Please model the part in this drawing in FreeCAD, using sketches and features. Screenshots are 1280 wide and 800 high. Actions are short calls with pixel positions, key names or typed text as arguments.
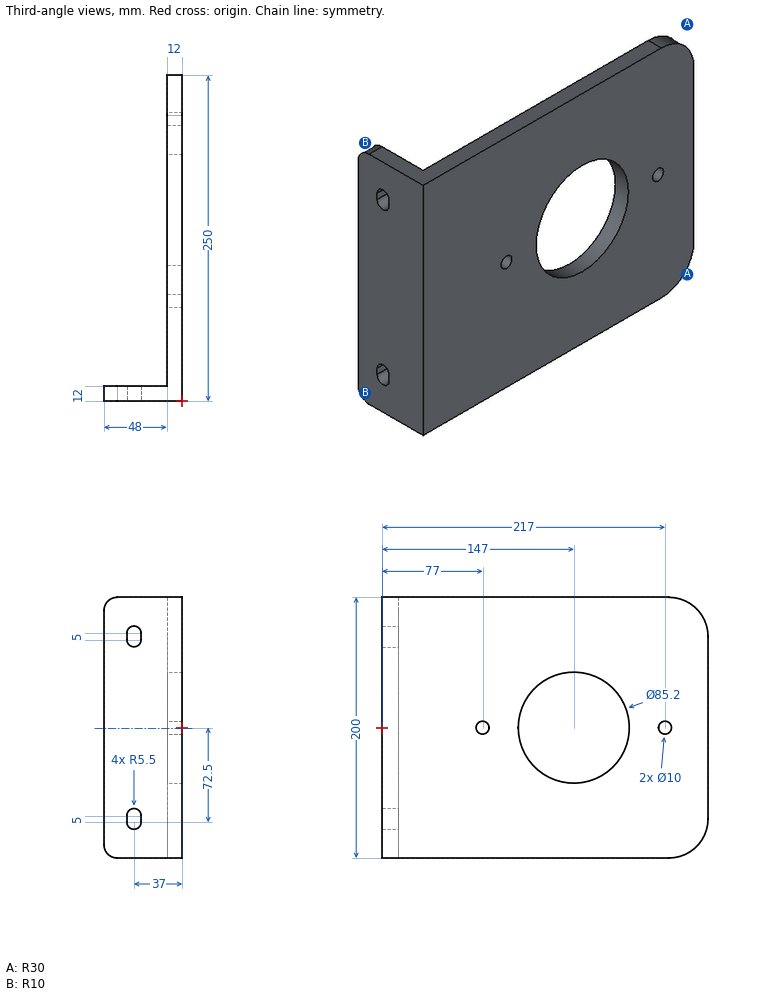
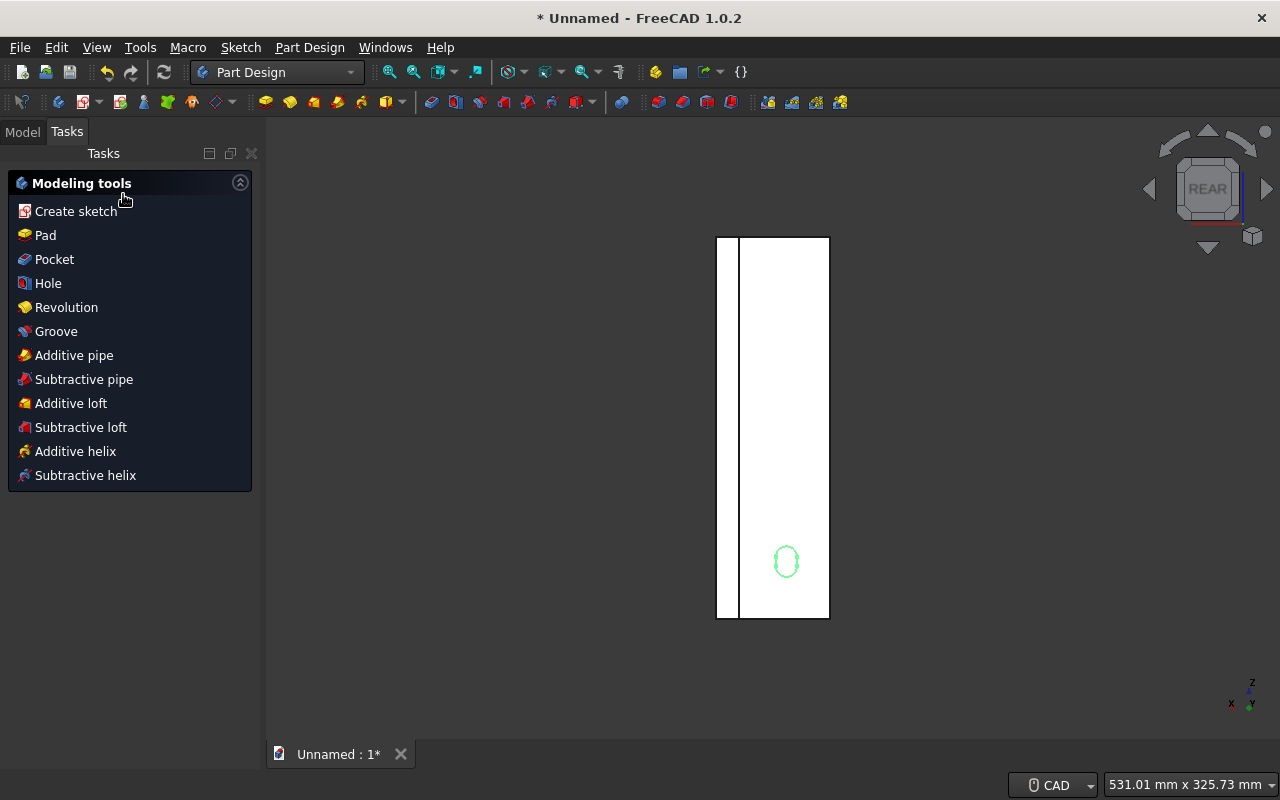
click(432, 102)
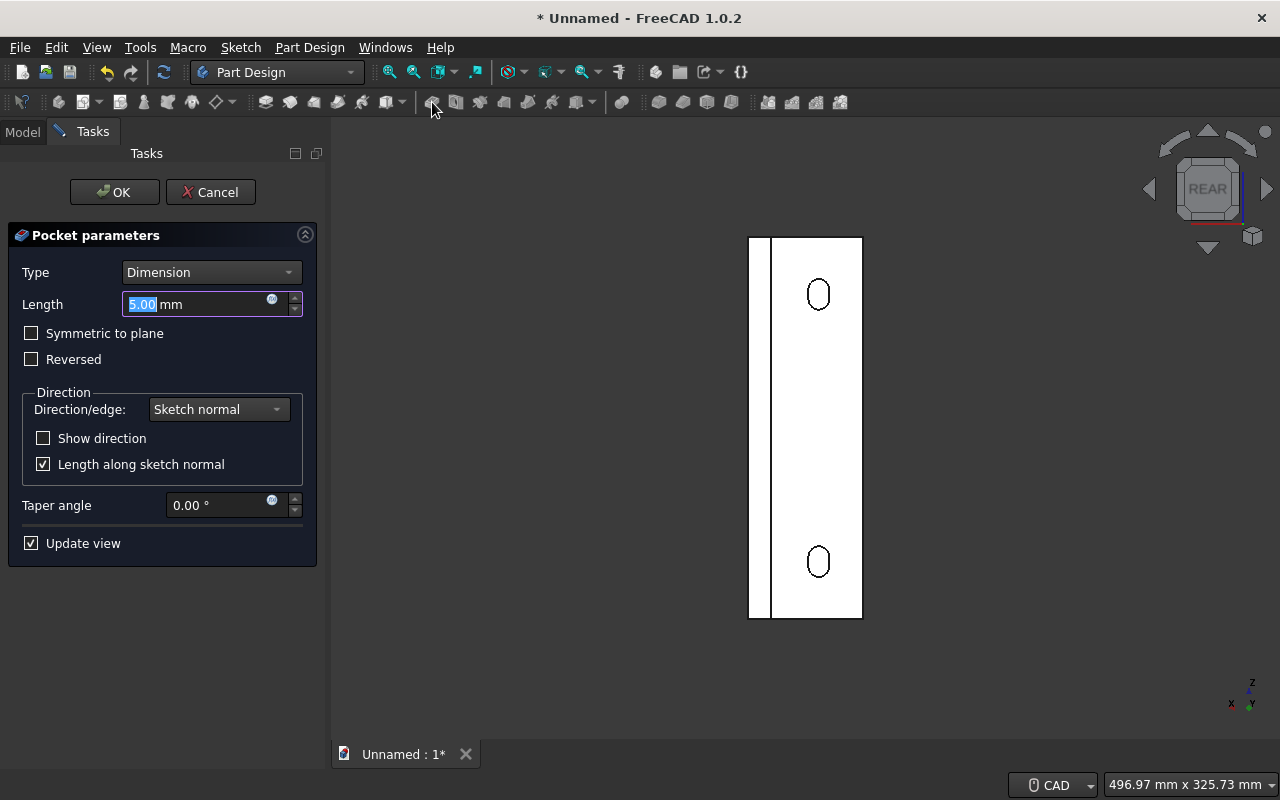
click(212, 272)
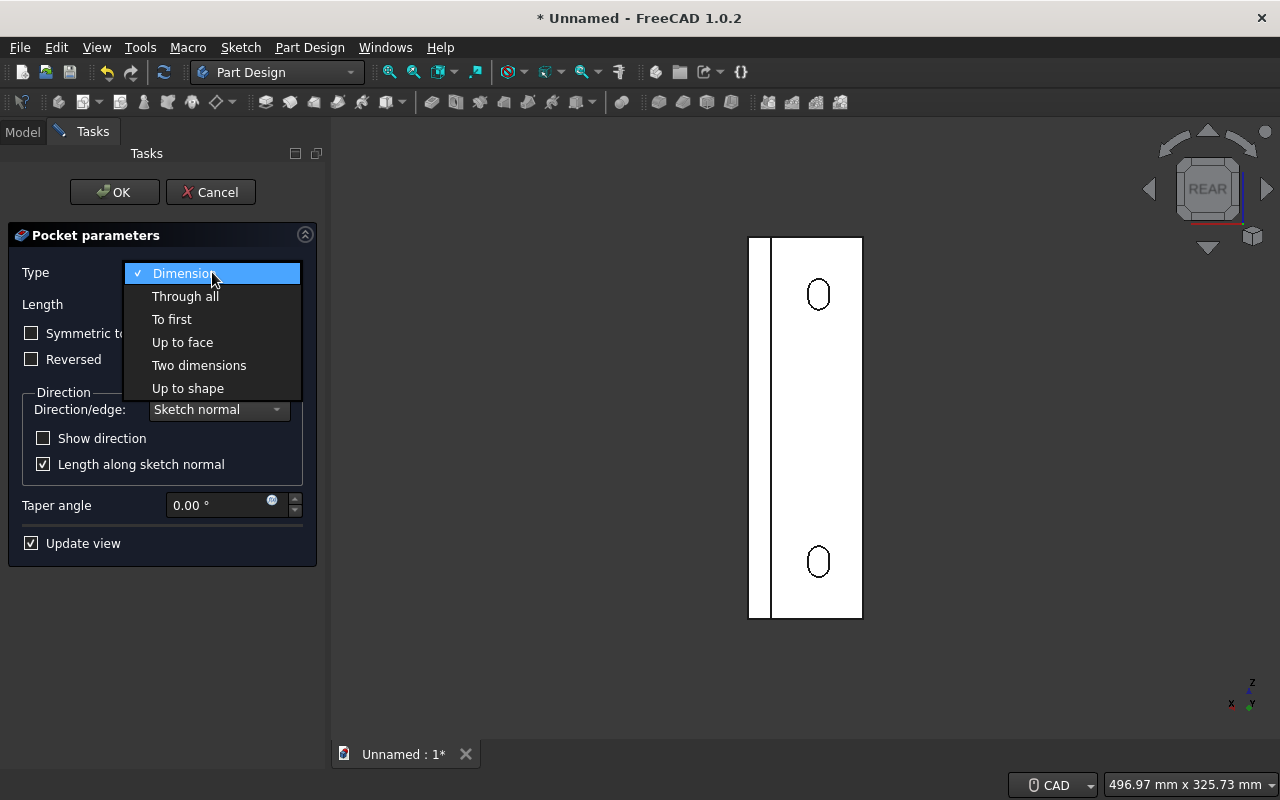
click(212, 296)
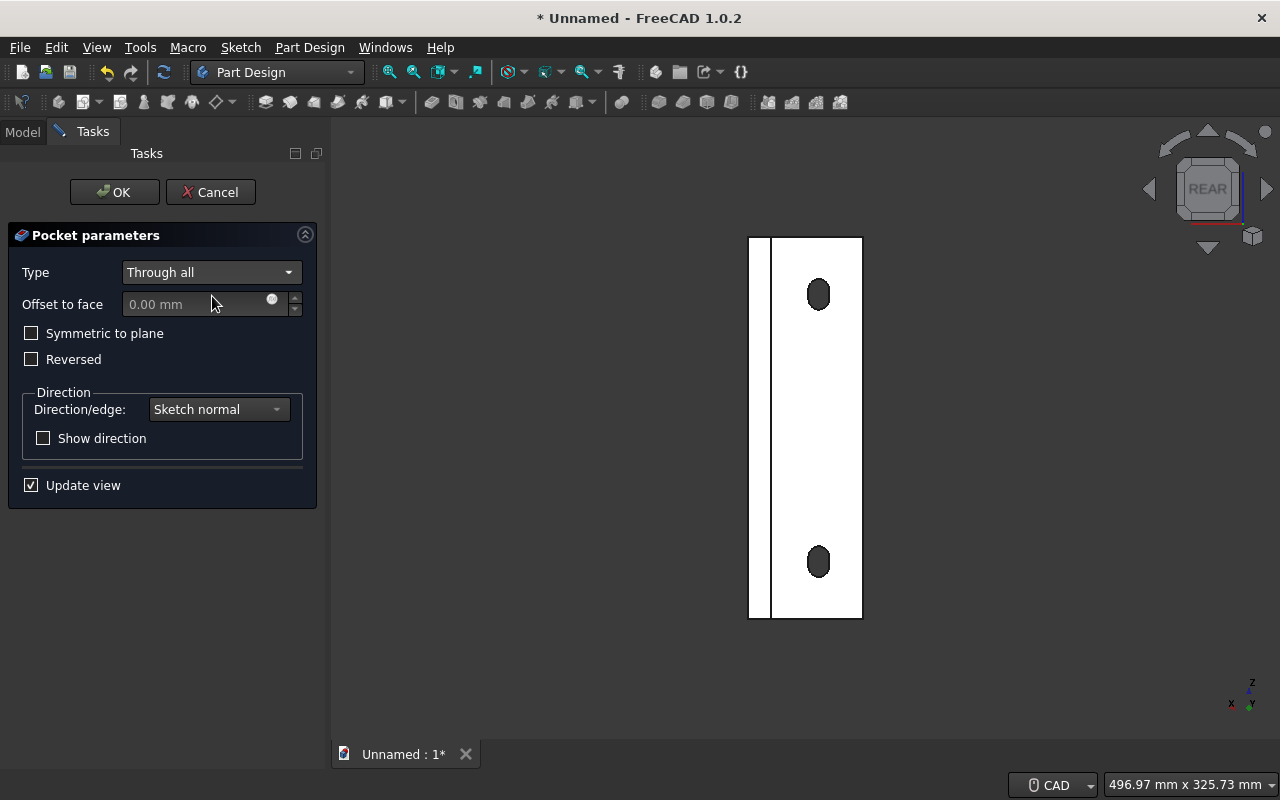
click(115, 192)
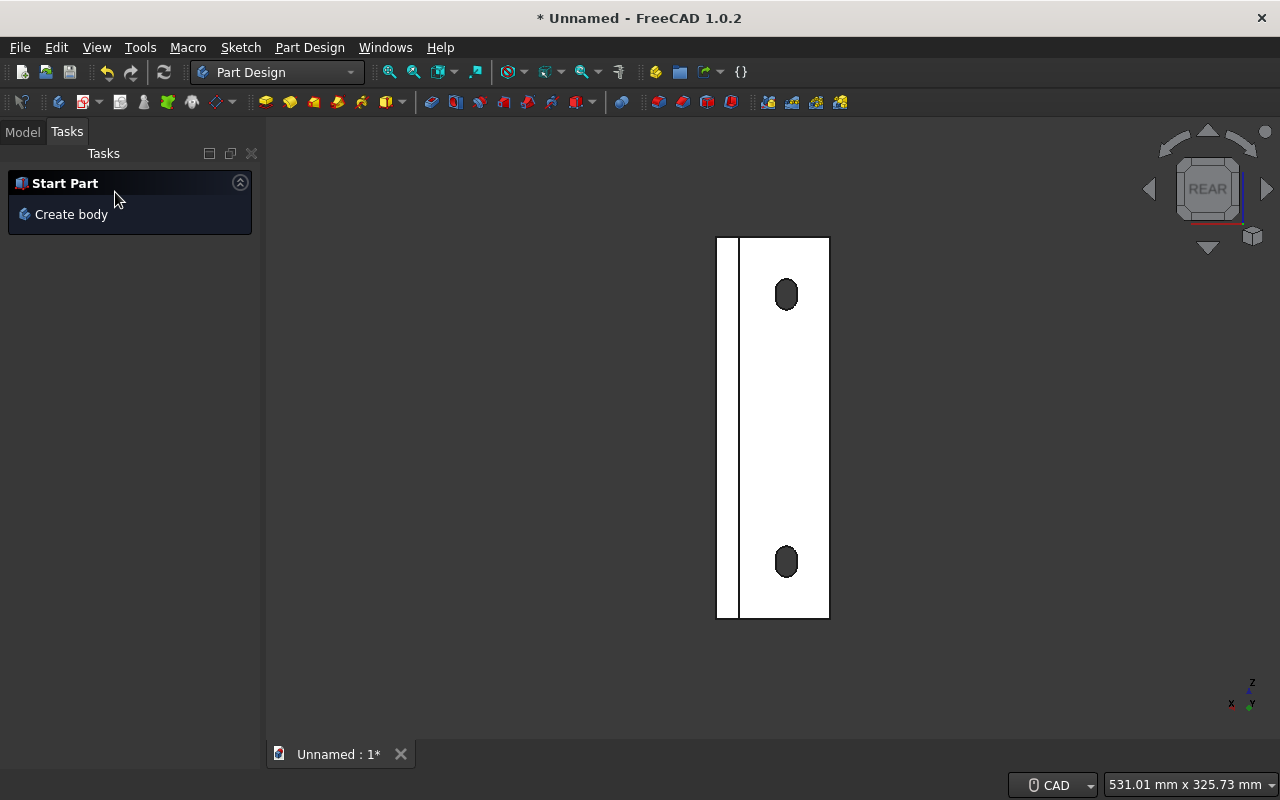
key(6)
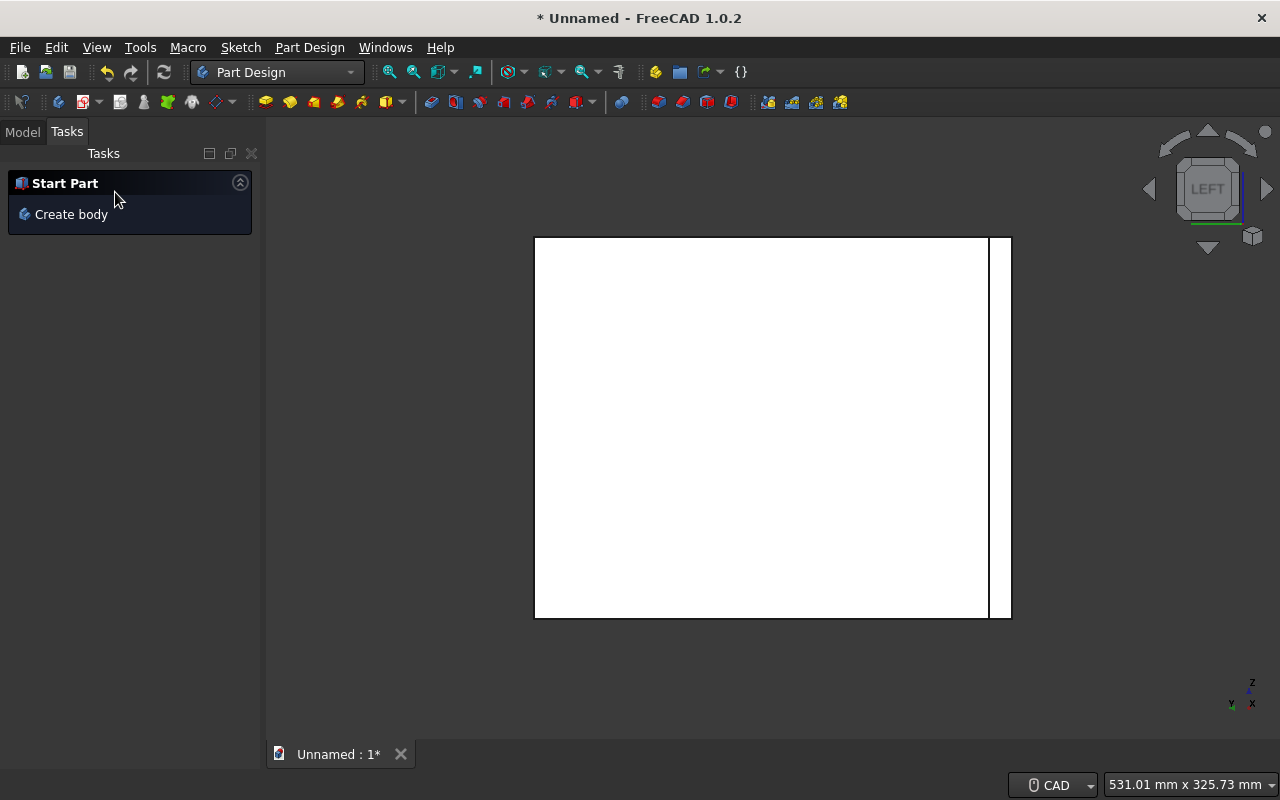
click(762, 427)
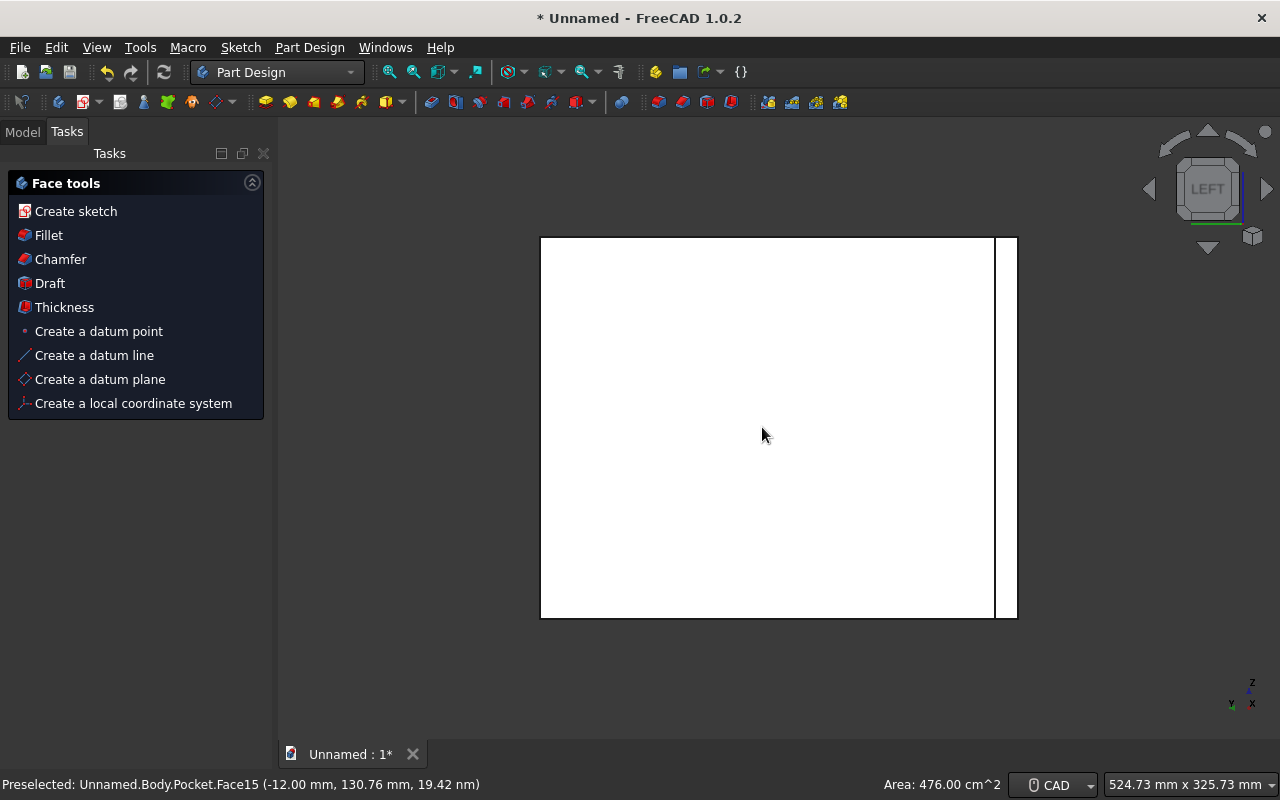
click(84, 102)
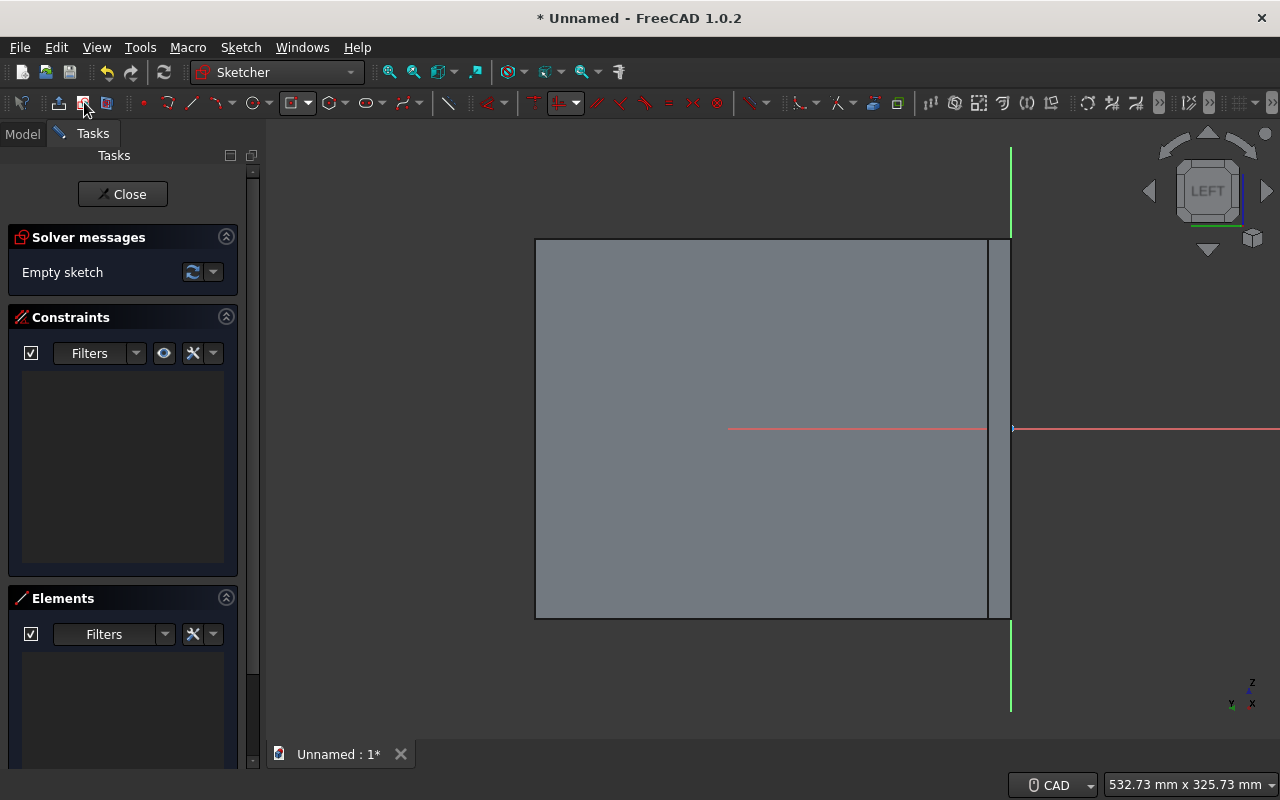
key(q)
key(s)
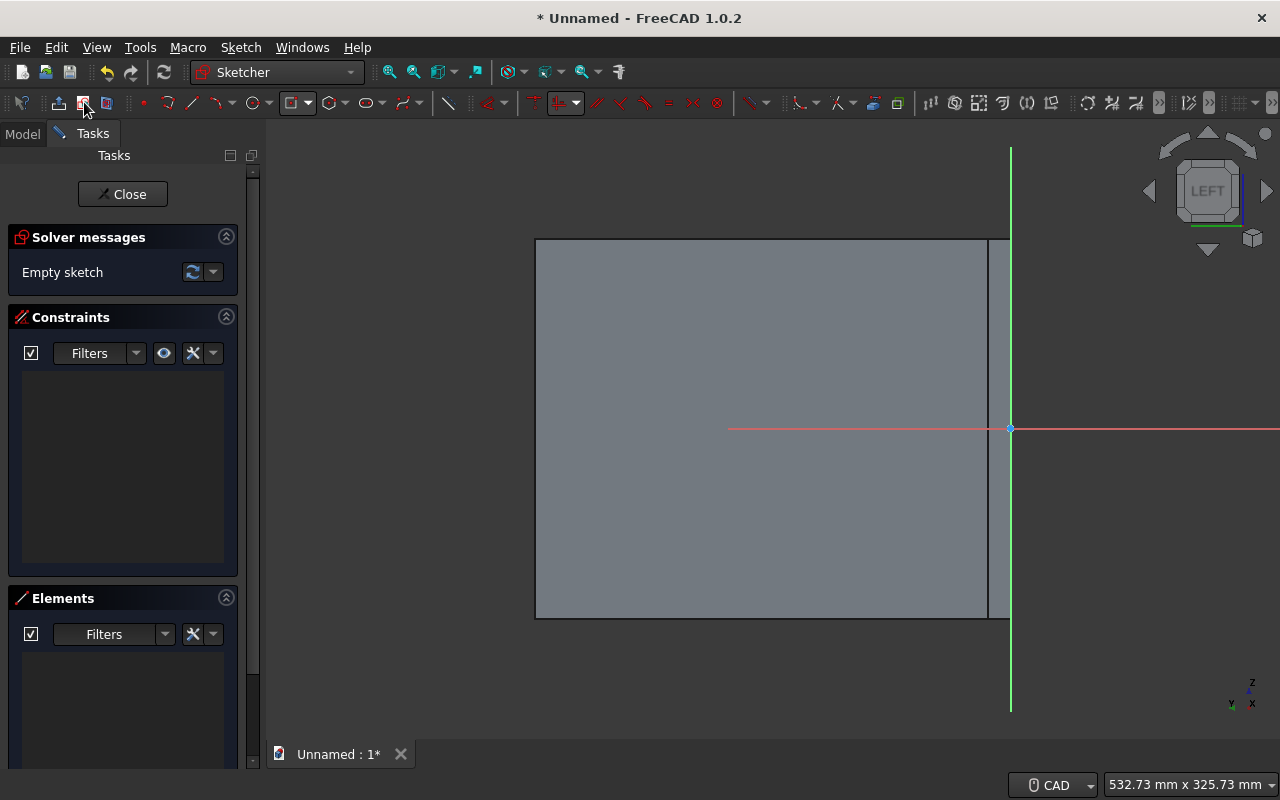
scroll(993, 429, up, 2)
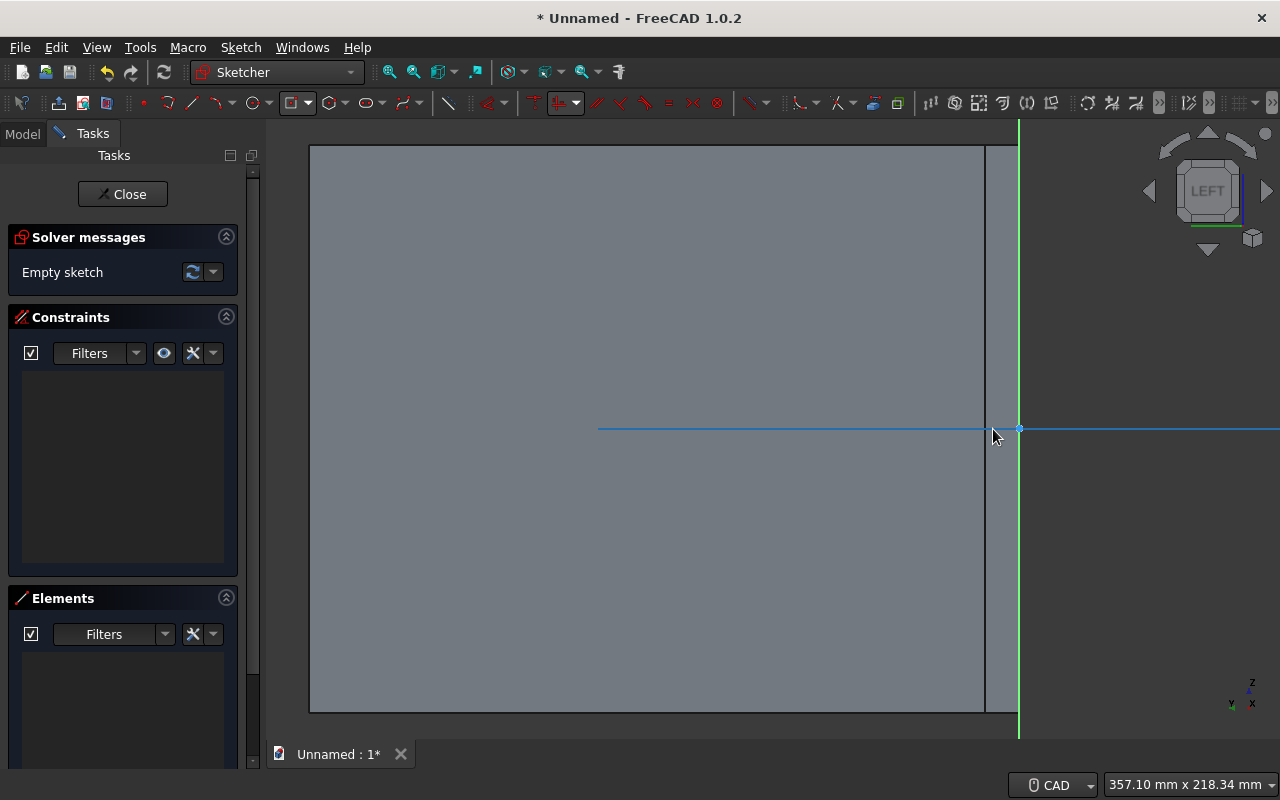
key(g)
key(c)